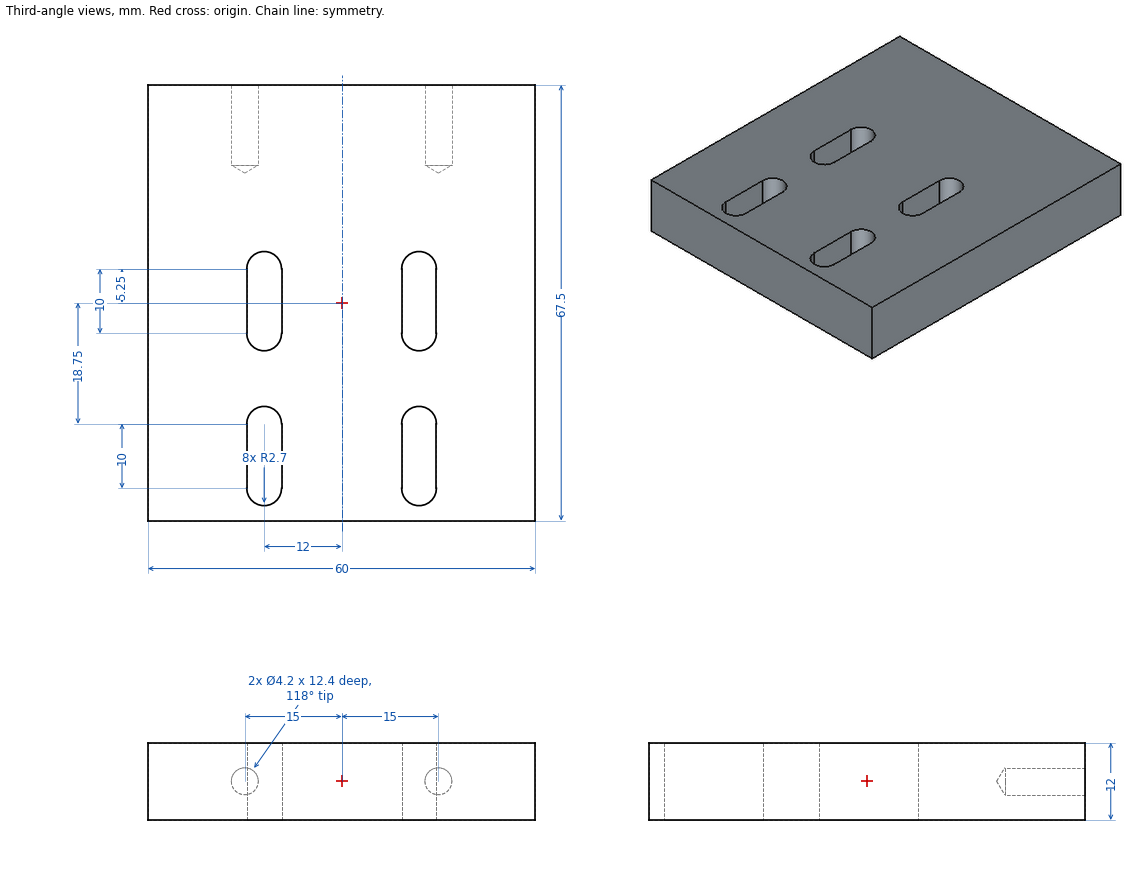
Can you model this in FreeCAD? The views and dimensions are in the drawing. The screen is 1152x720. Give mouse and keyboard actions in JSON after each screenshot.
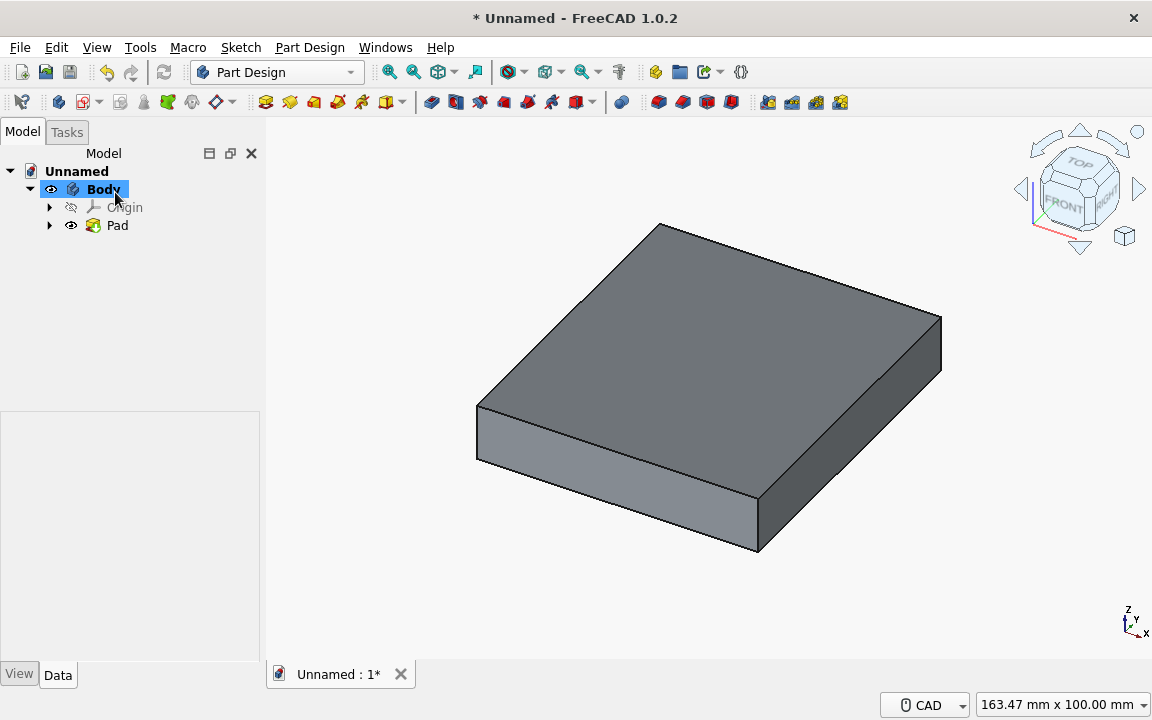
{"action": "key", "text": "5"}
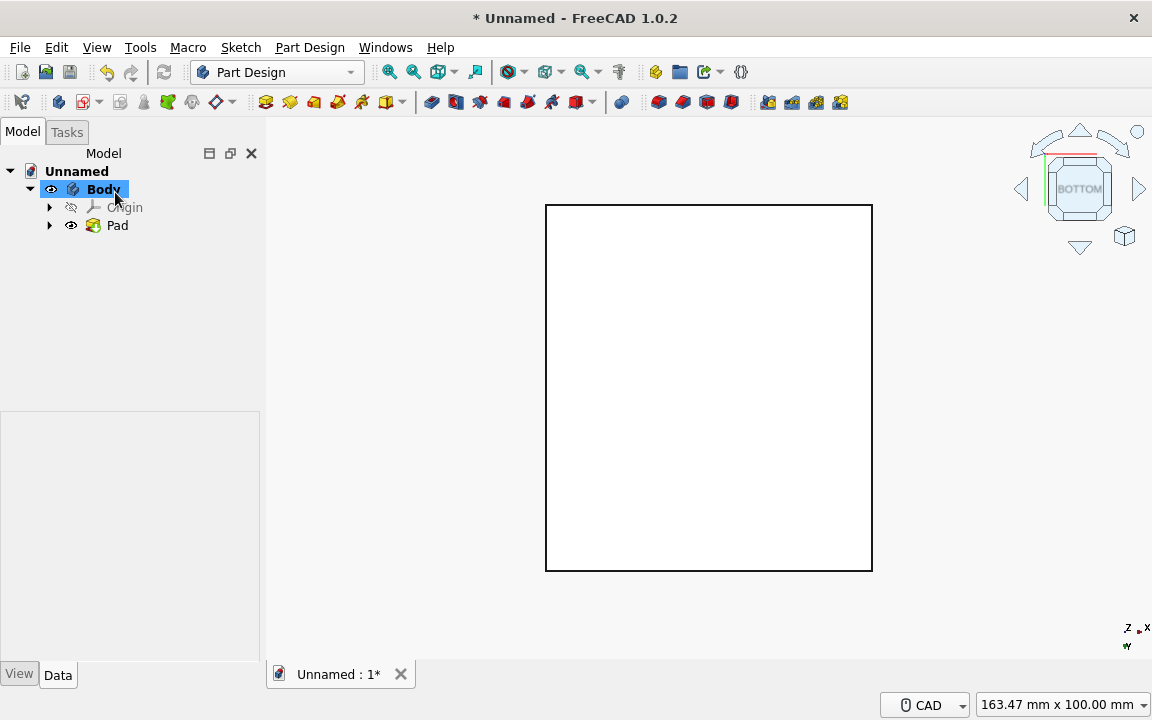
{"action": "left_click", "coordinate": [709, 387]}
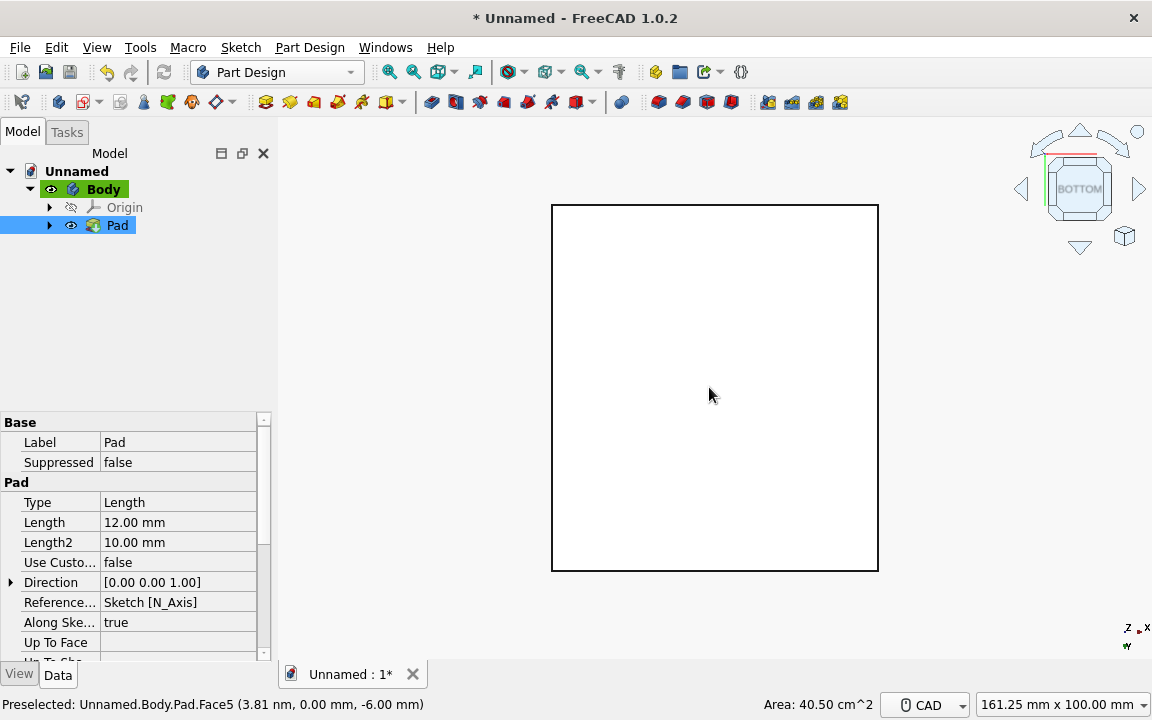
{"action": "left_click", "coordinate": [84, 102]}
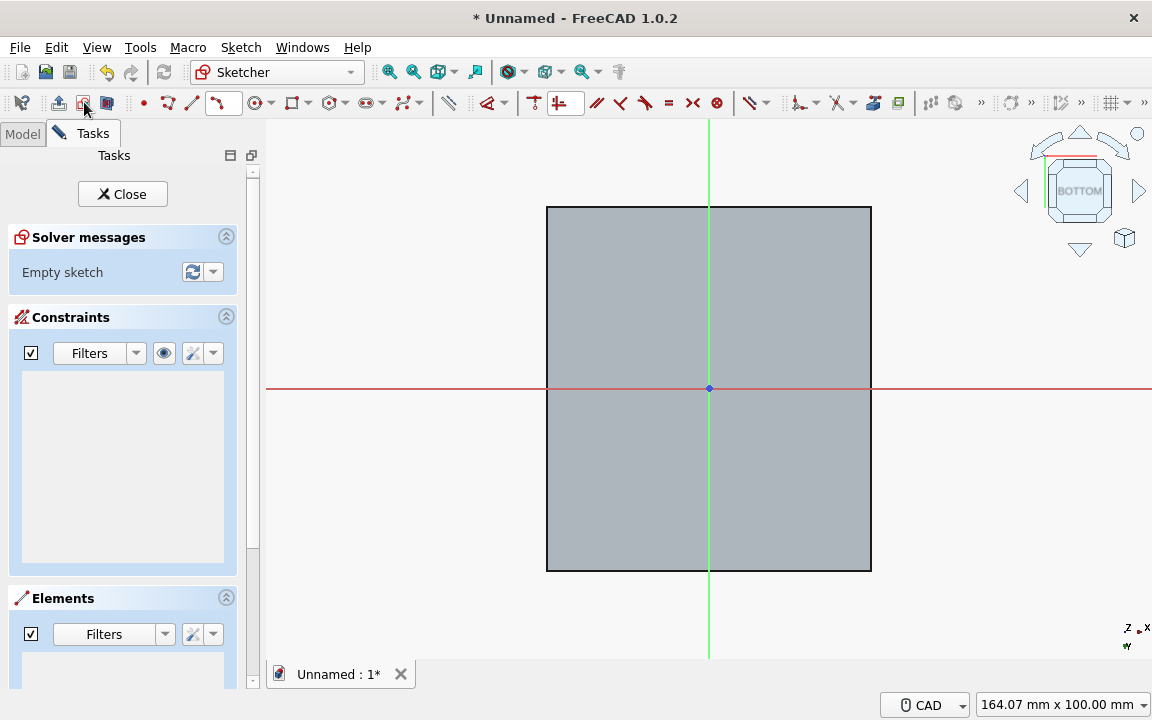
{"action": "scroll", "coordinate": [848, 197], "scroll_direction": "up", "scroll_amount": 2}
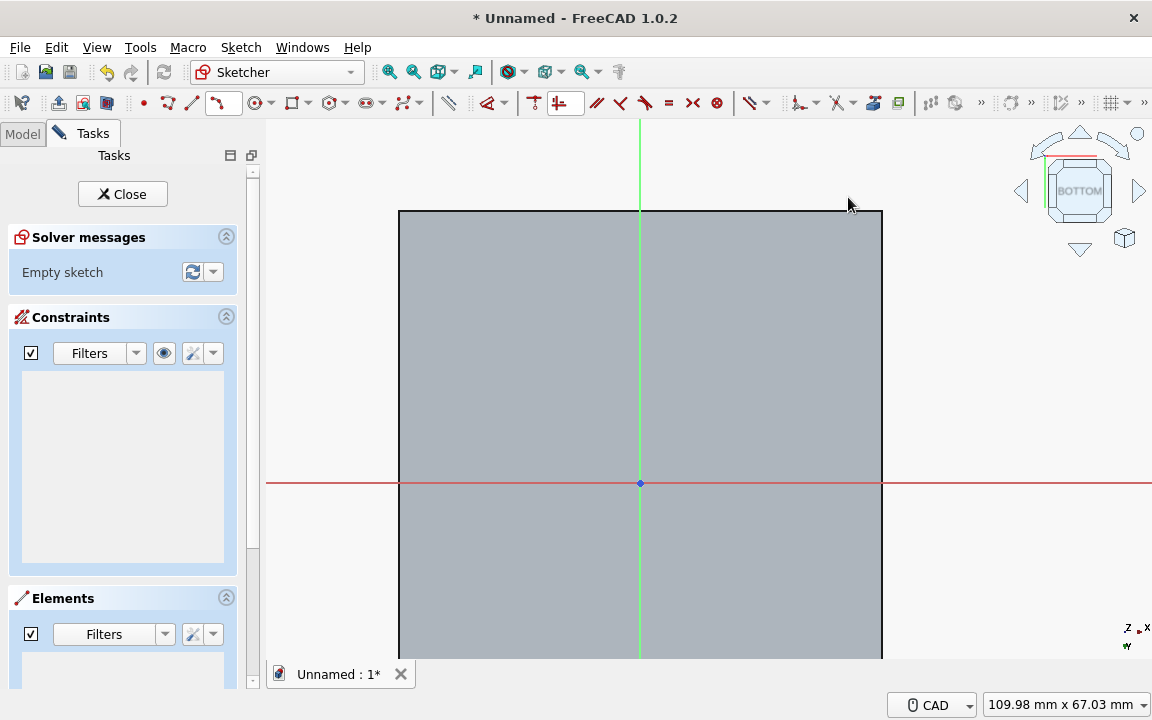
{"action": "key", "text": "g s"}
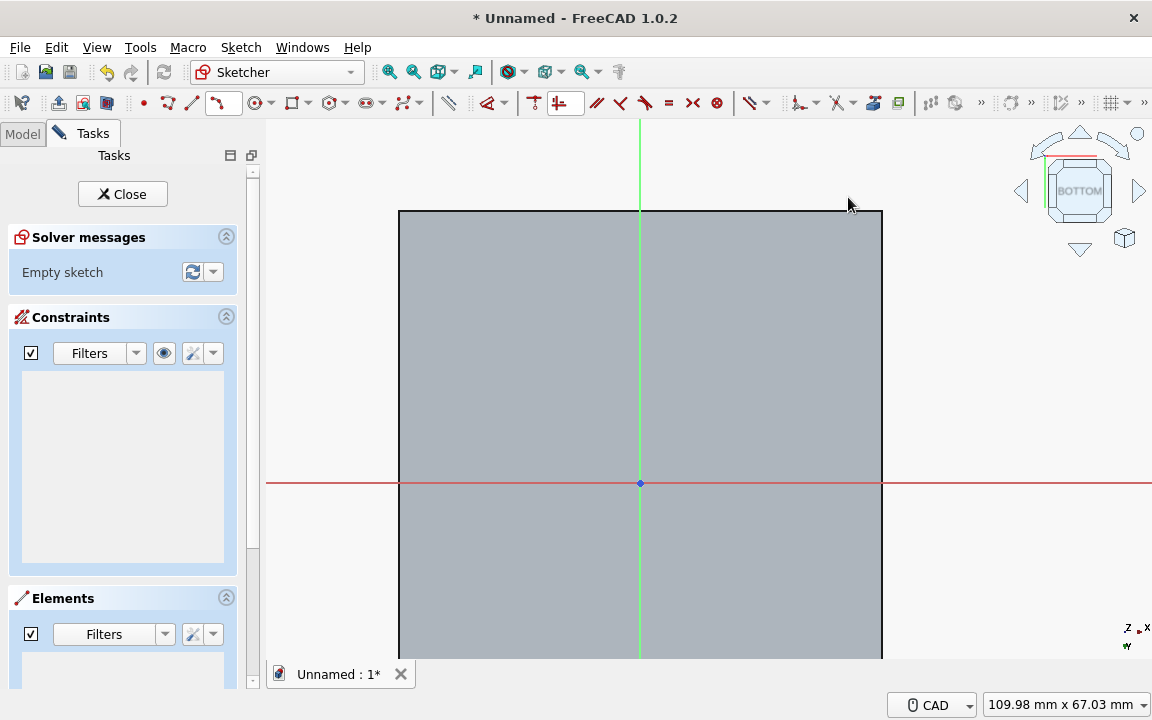
{"action": "left_click", "coordinate": [544, 332]}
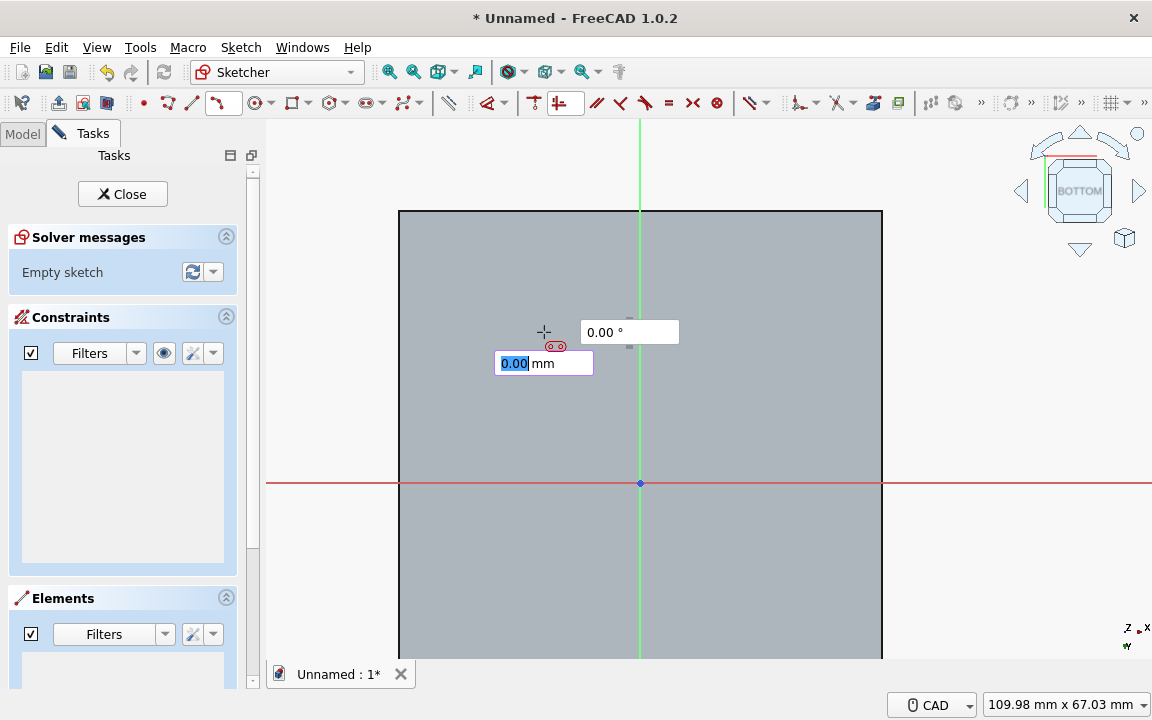
{"action": "left_click", "coordinate": [544, 252]}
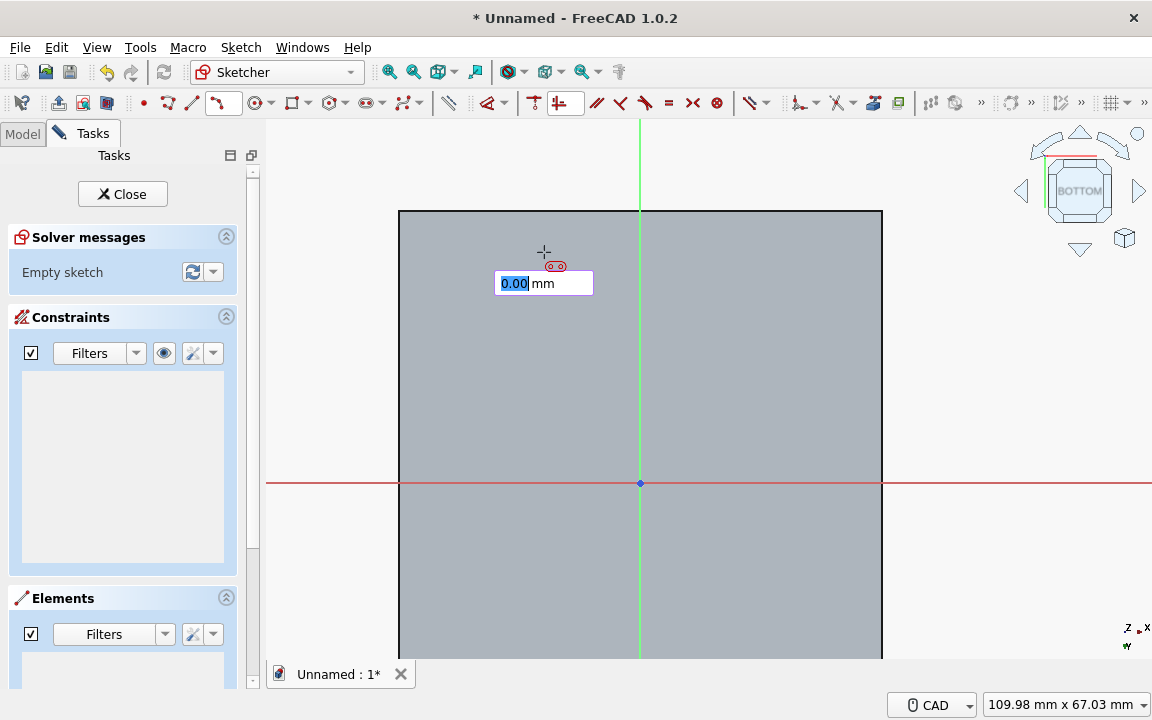
{"action": "left_click", "coordinate": [565, 292]}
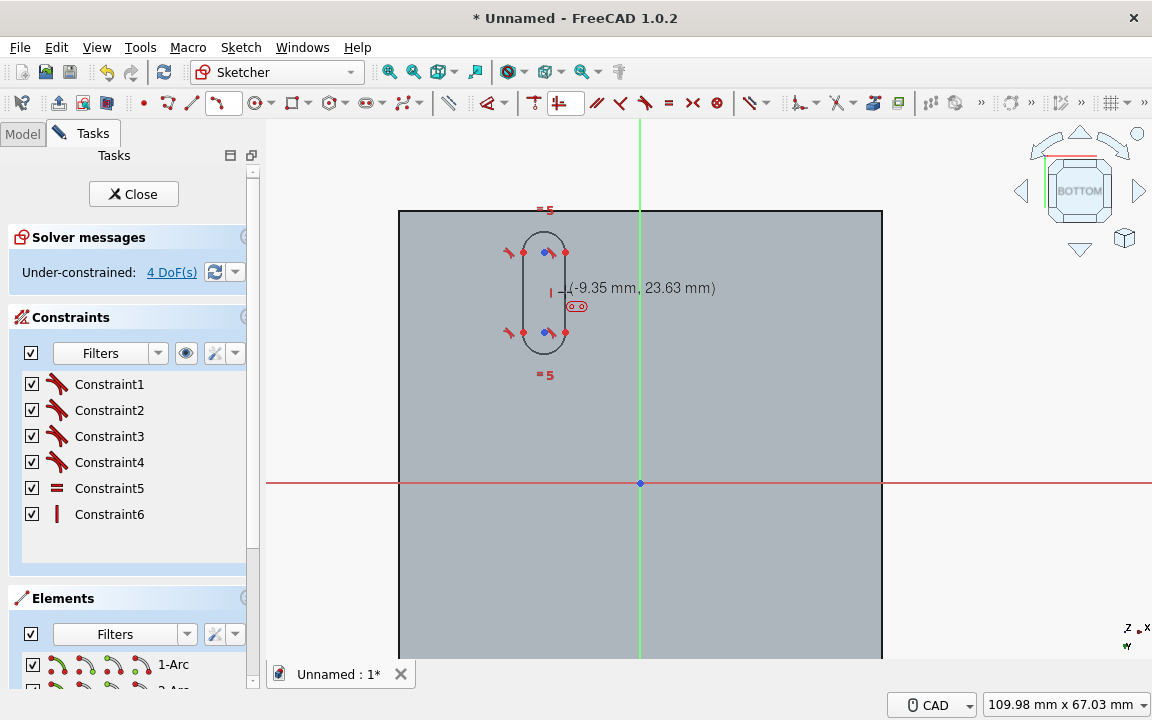
{"action": "left_click", "coordinate": [737, 332]}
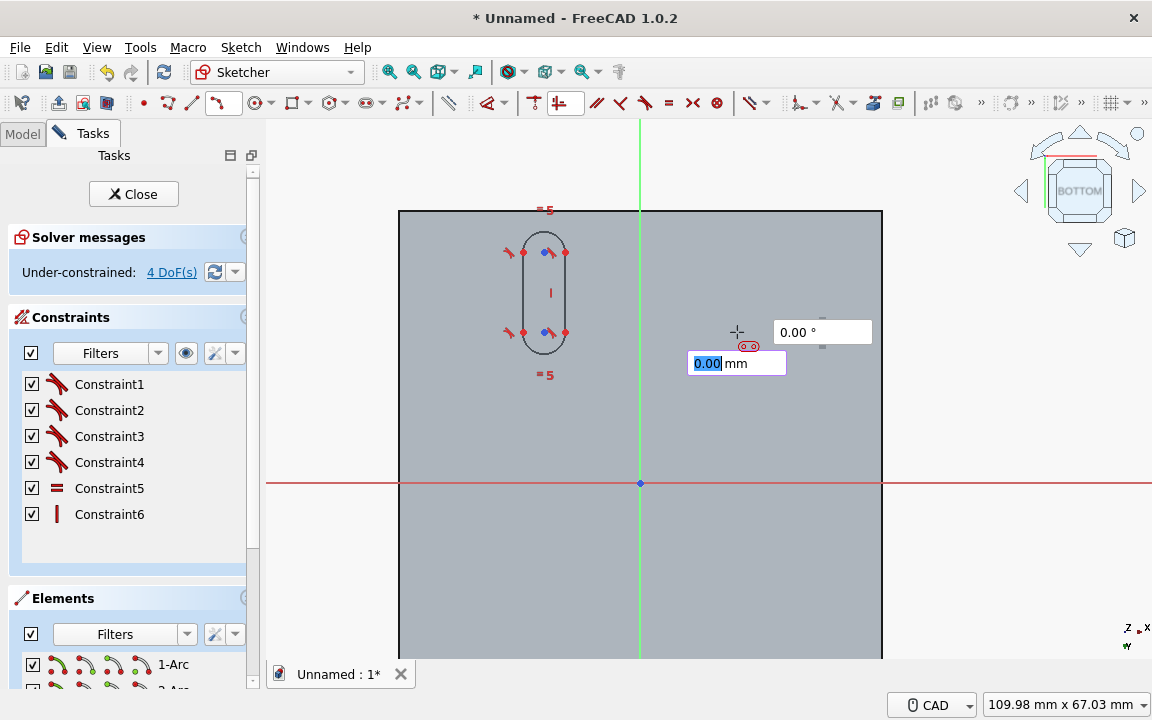
{"action": "left_click", "coordinate": [737, 252]}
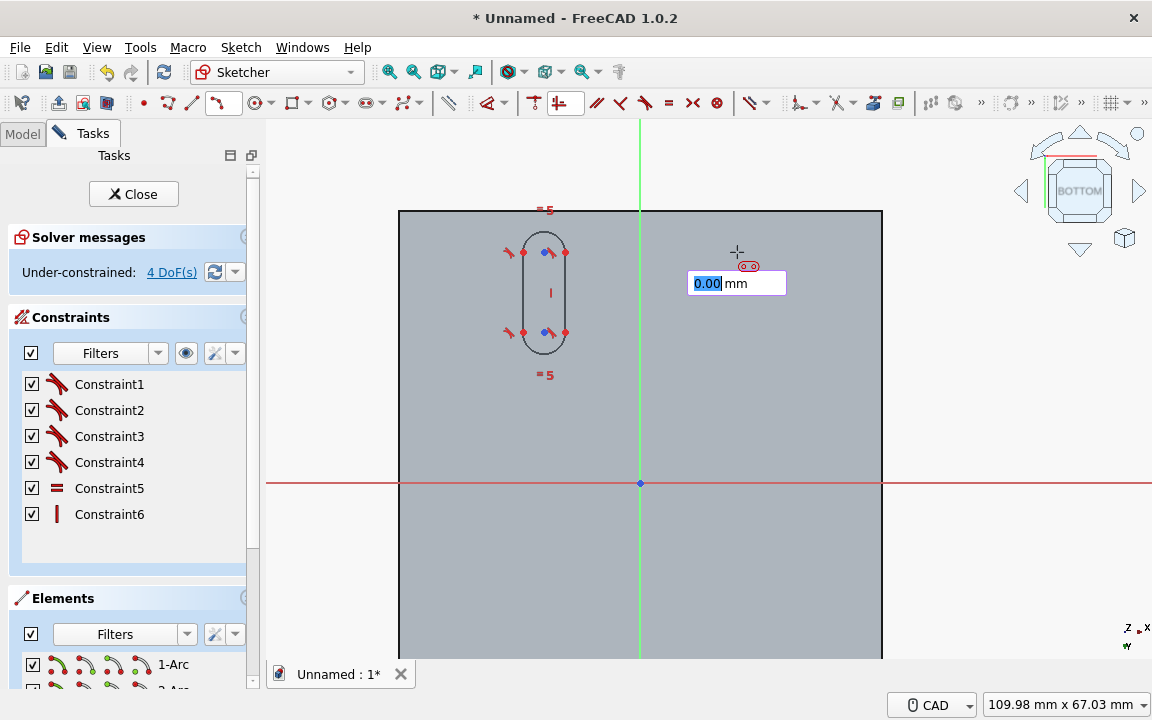
{"action": "left_click", "coordinate": [759, 292]}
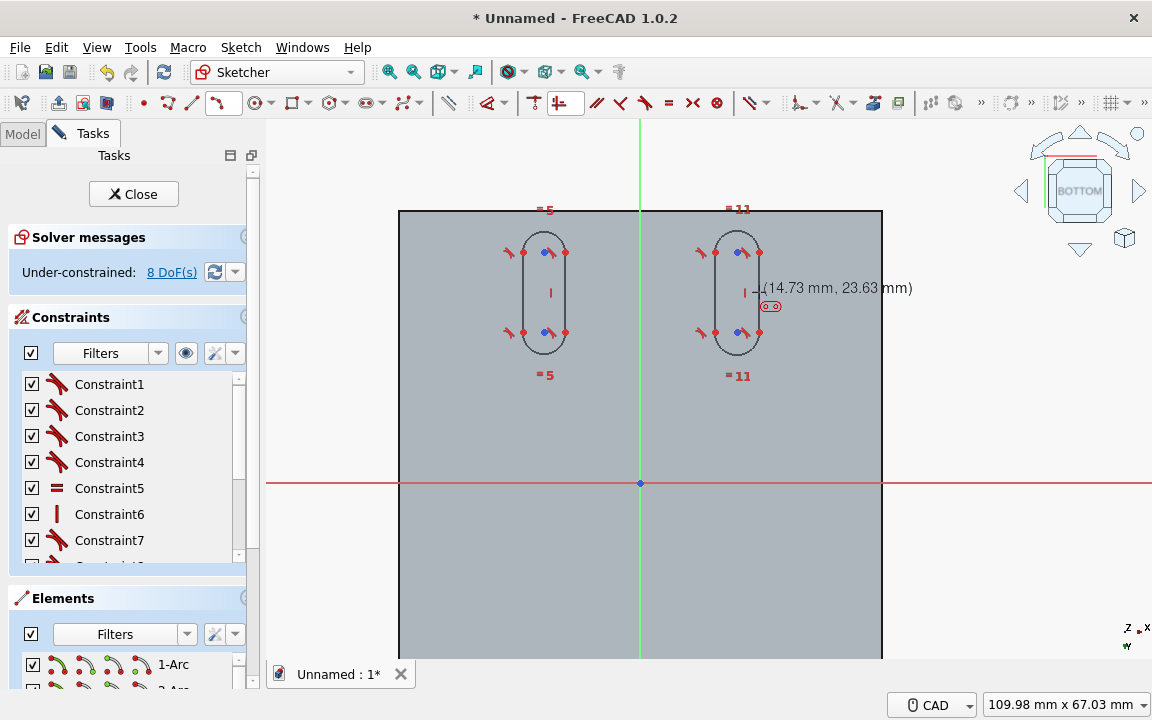
{"action": "left_click", "coordinate": [544, 526]}